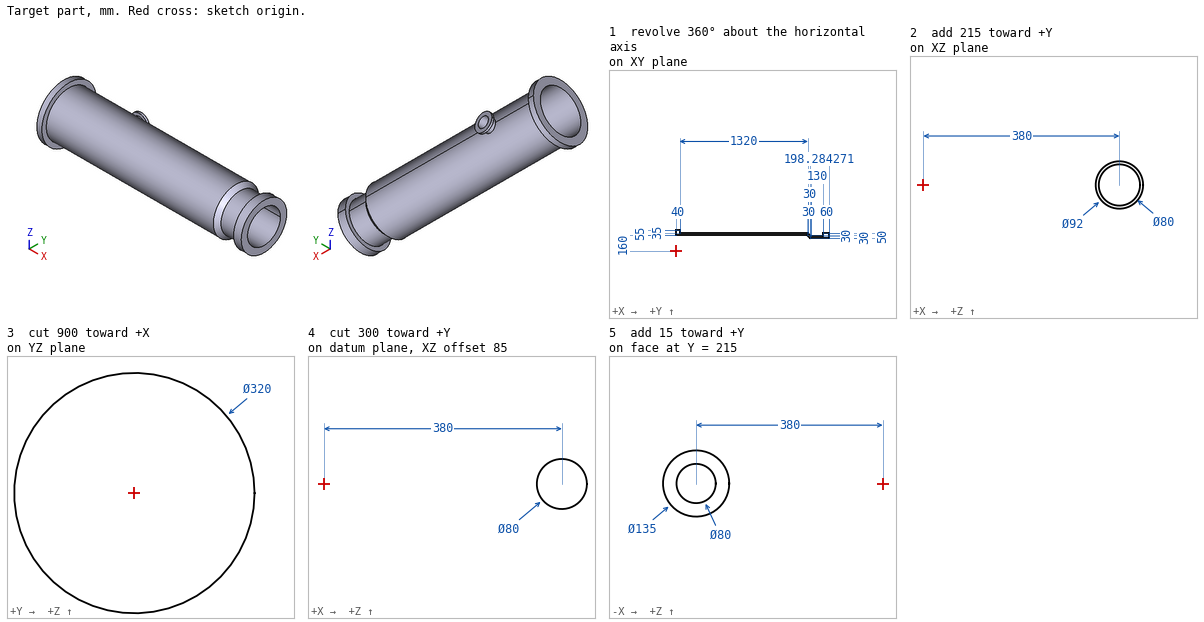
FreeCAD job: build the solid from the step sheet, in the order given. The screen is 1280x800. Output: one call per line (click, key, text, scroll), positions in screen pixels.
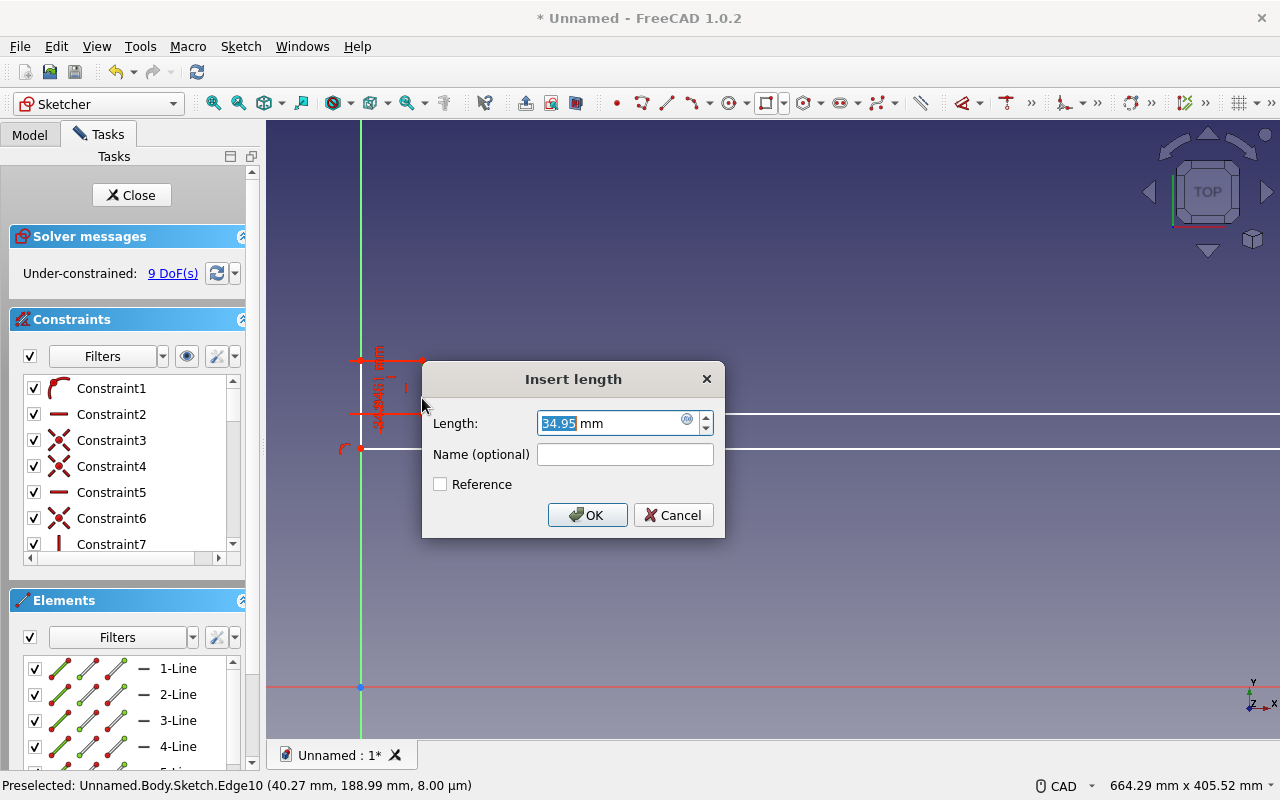
text(35)
key(Return)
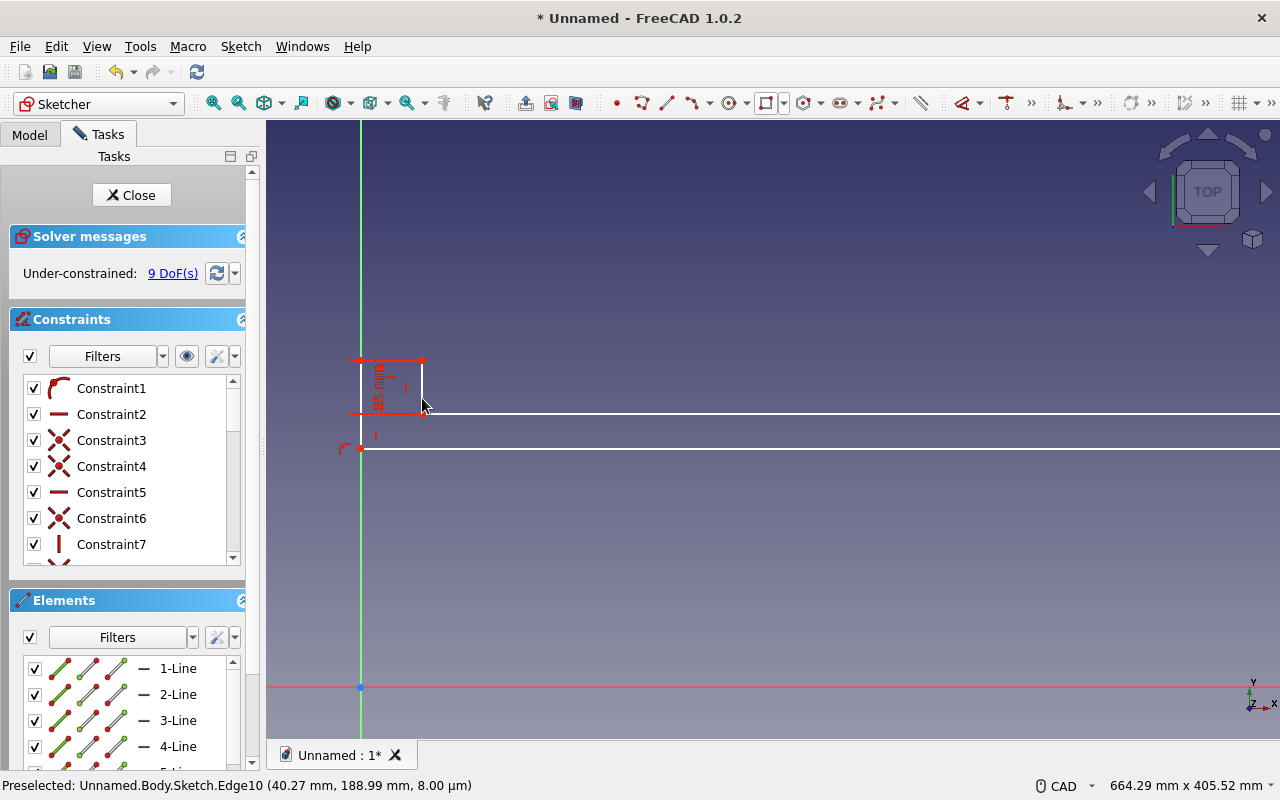
click(404, 361)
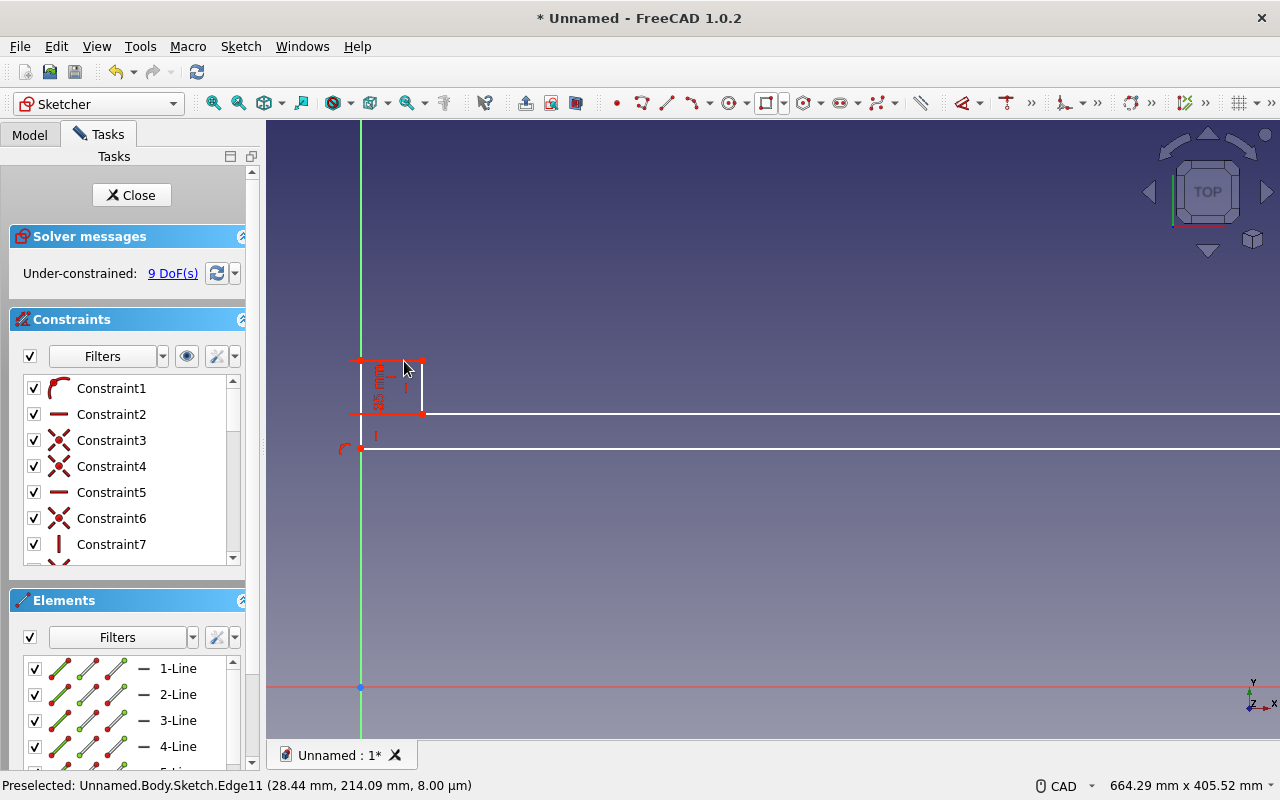
key(l)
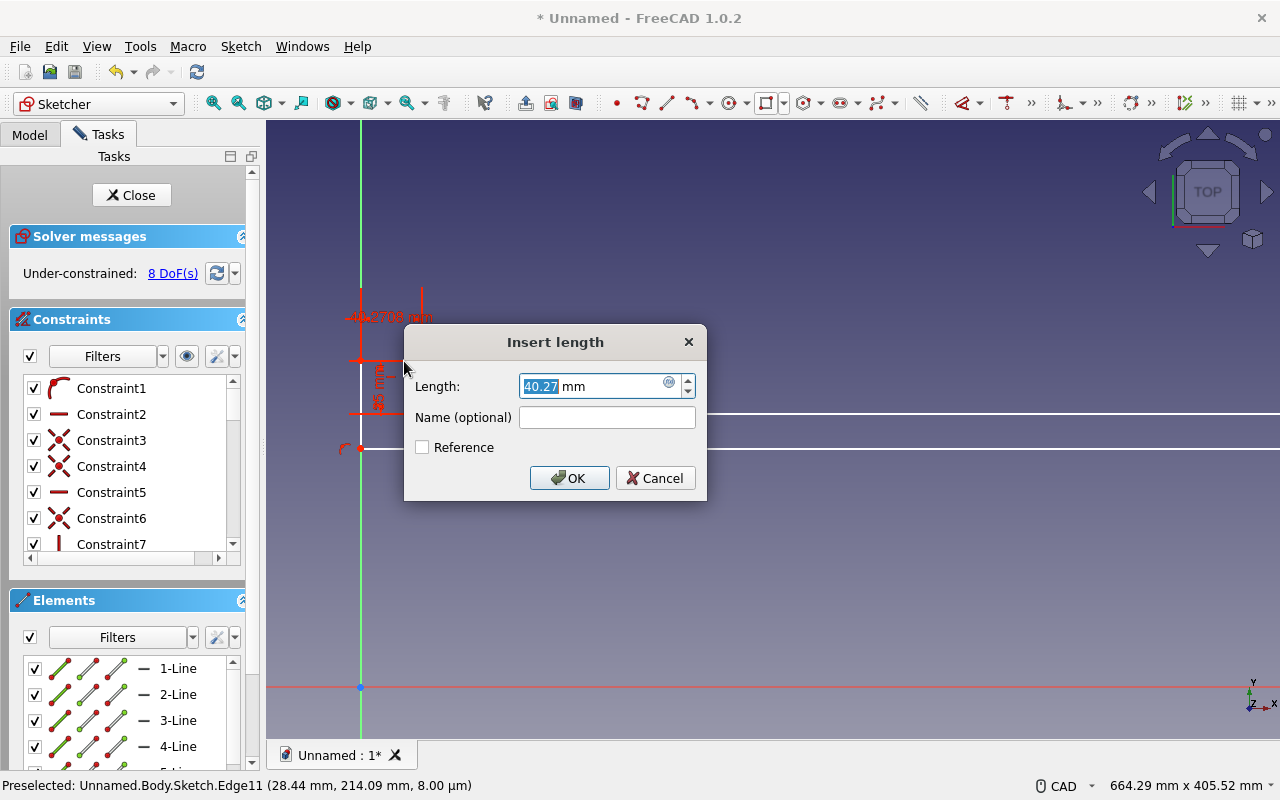
text(40)
key(Return)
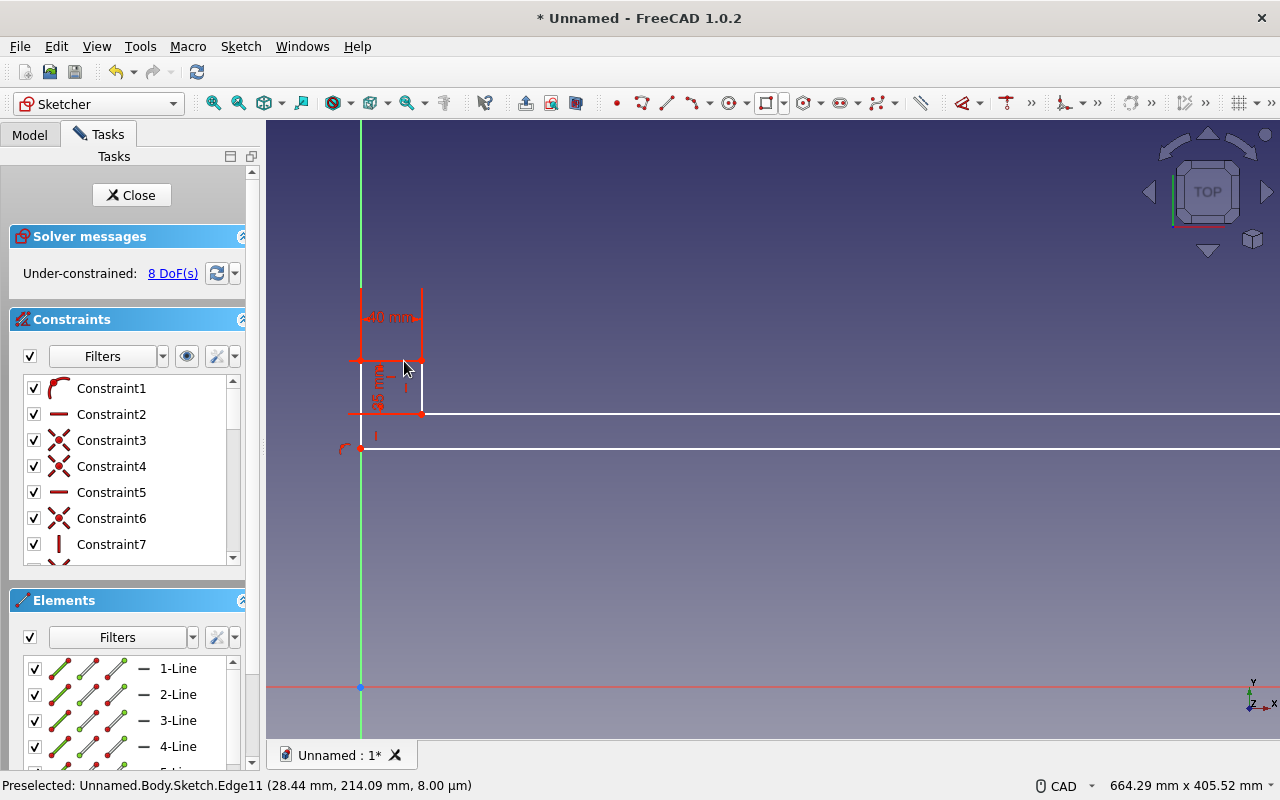
click(361, 387)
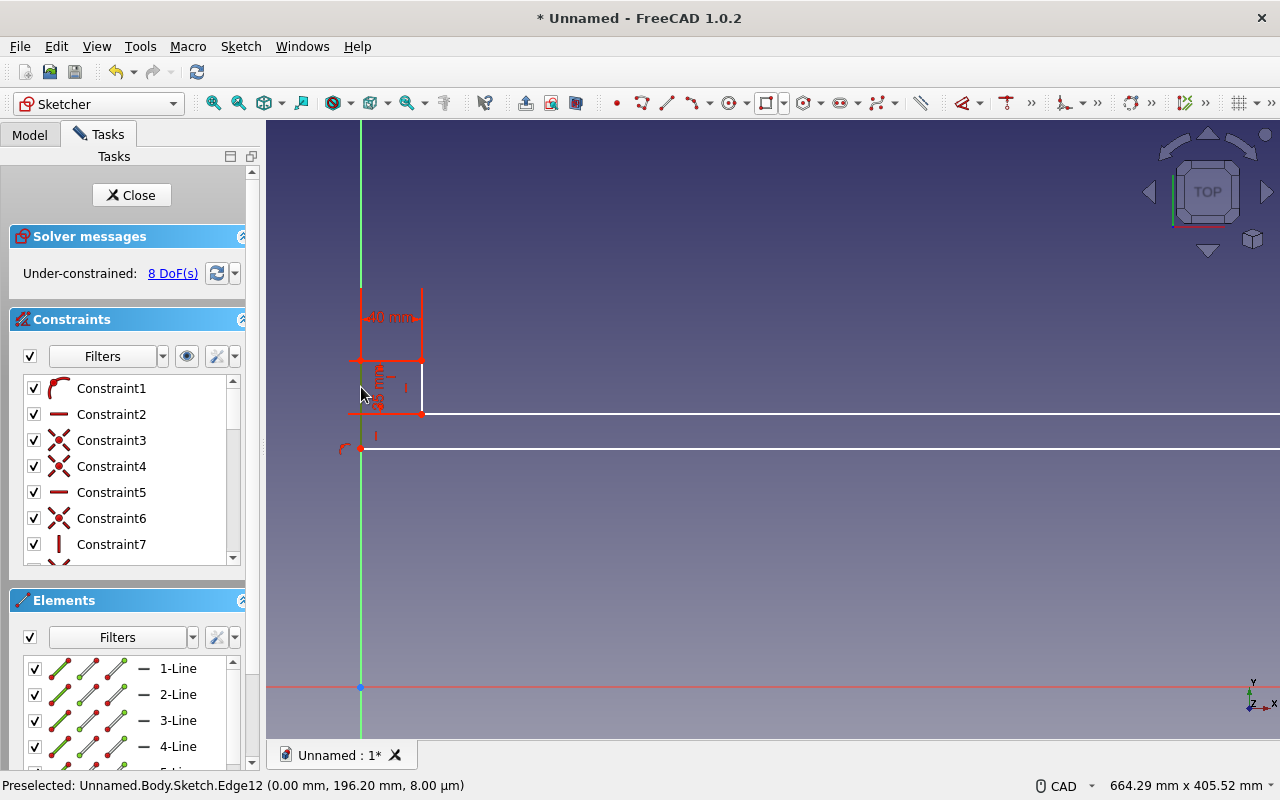
key(i)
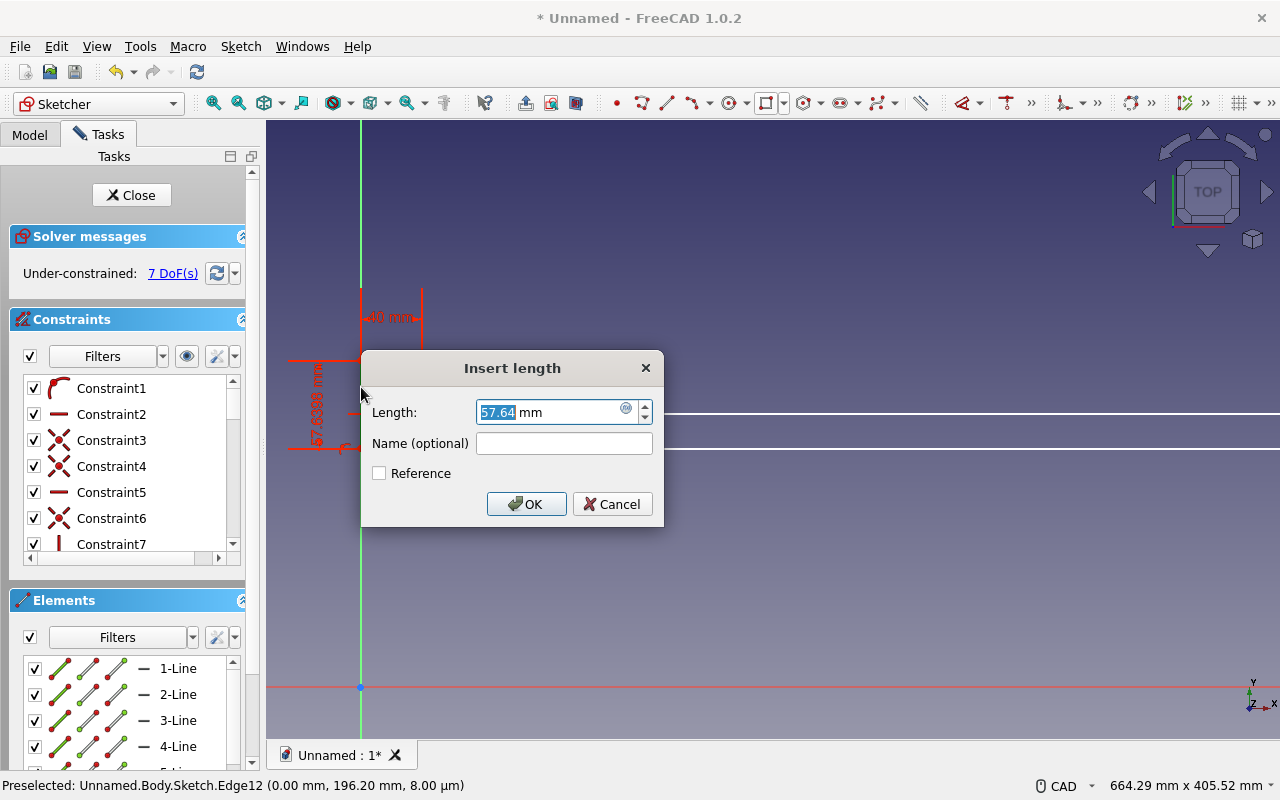
text(55)
key(Return)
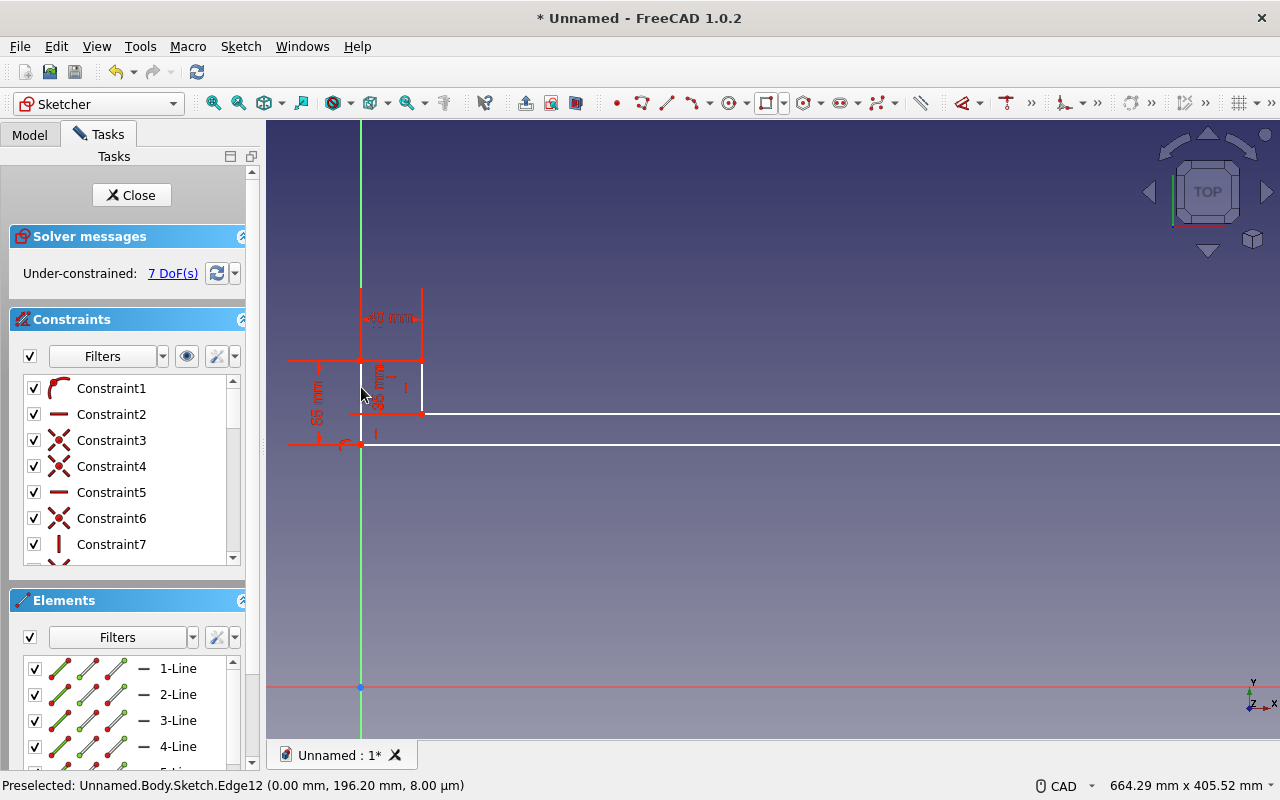
scroll(422, 399, down, 7)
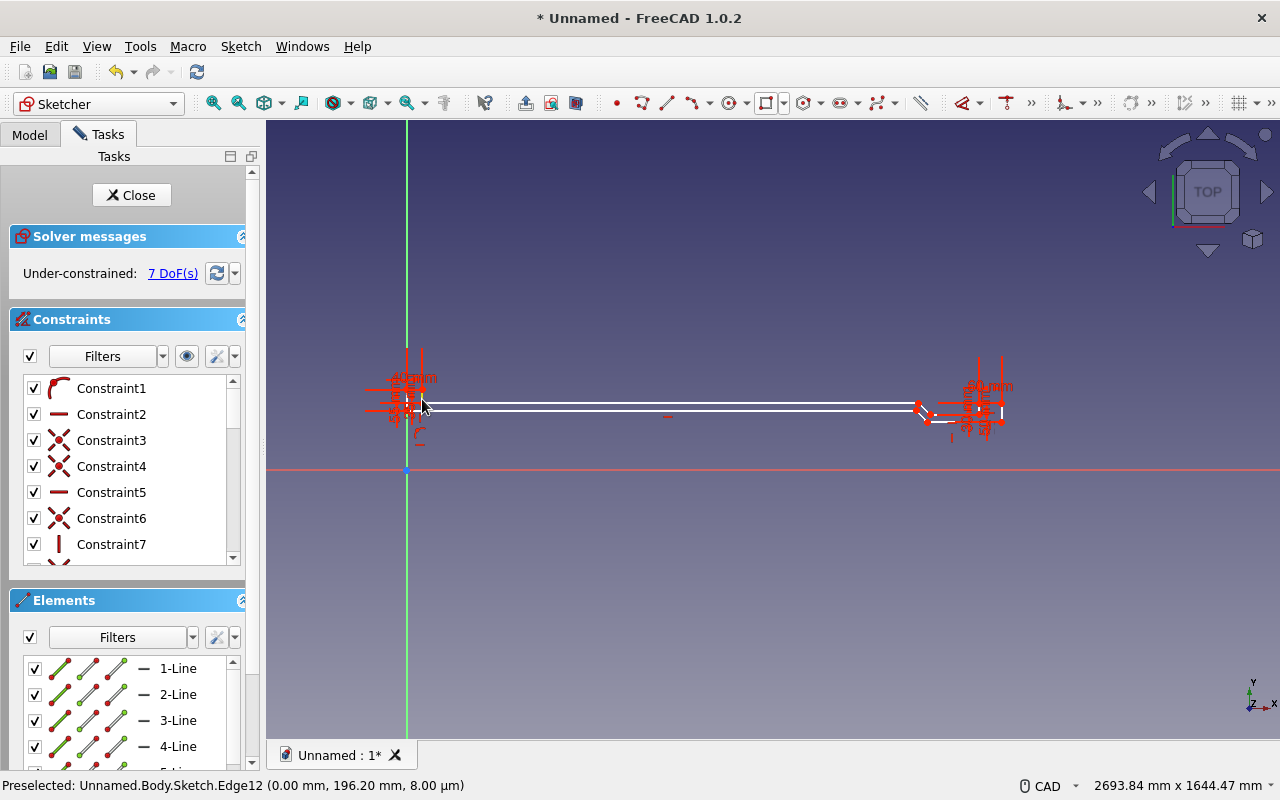
scroll(965, 415, up, 4)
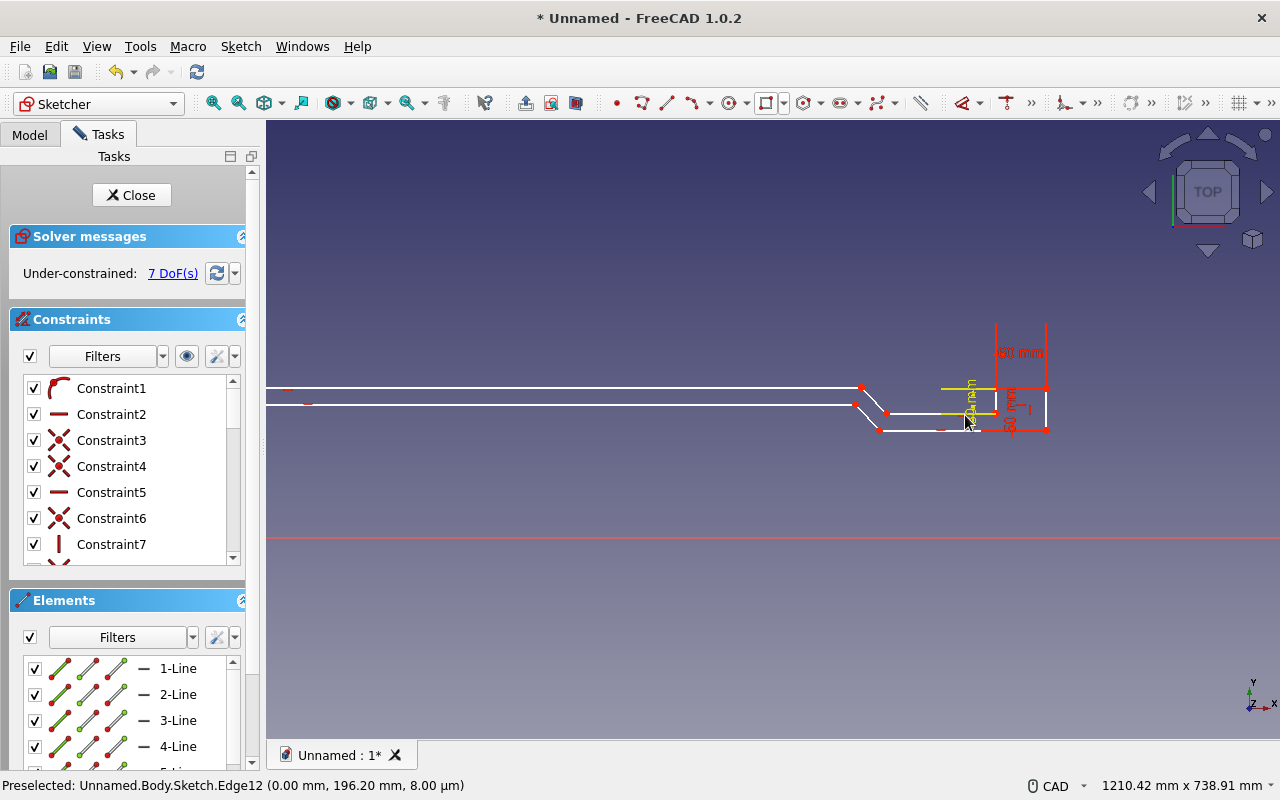
click(919, 414)